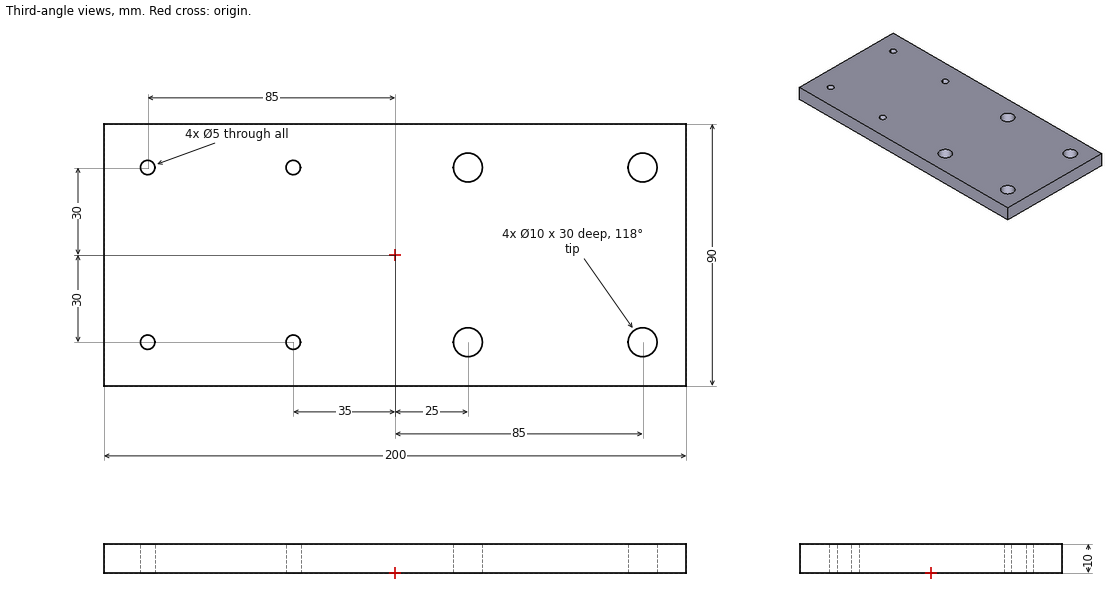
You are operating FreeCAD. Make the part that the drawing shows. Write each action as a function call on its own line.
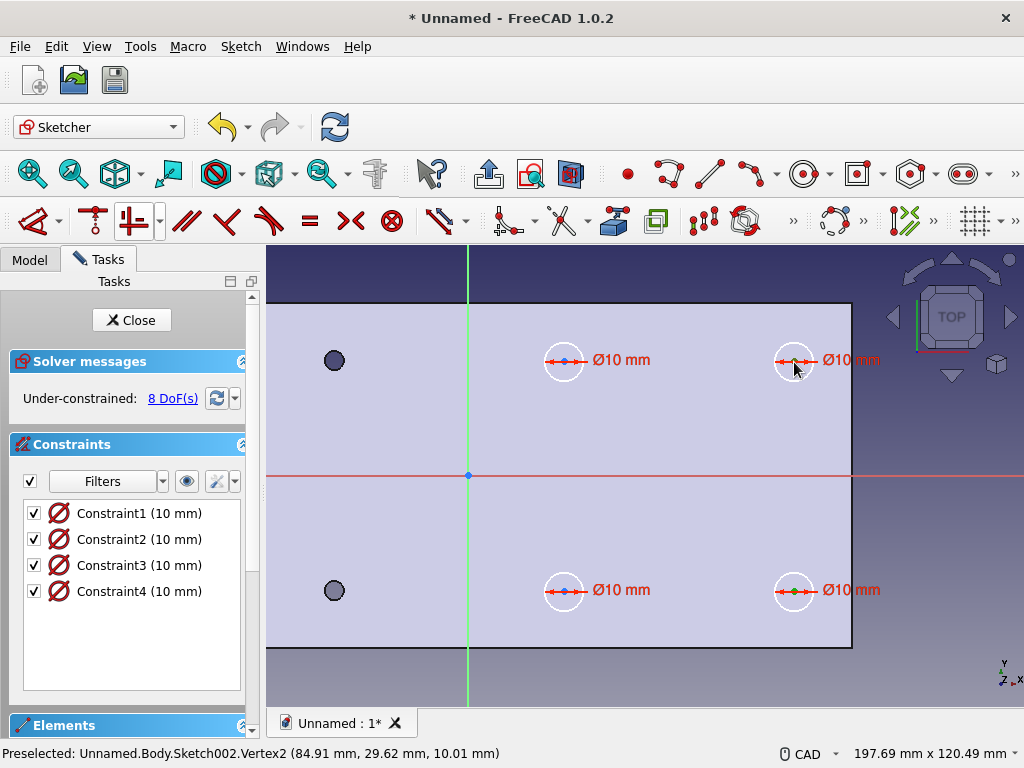
key(v)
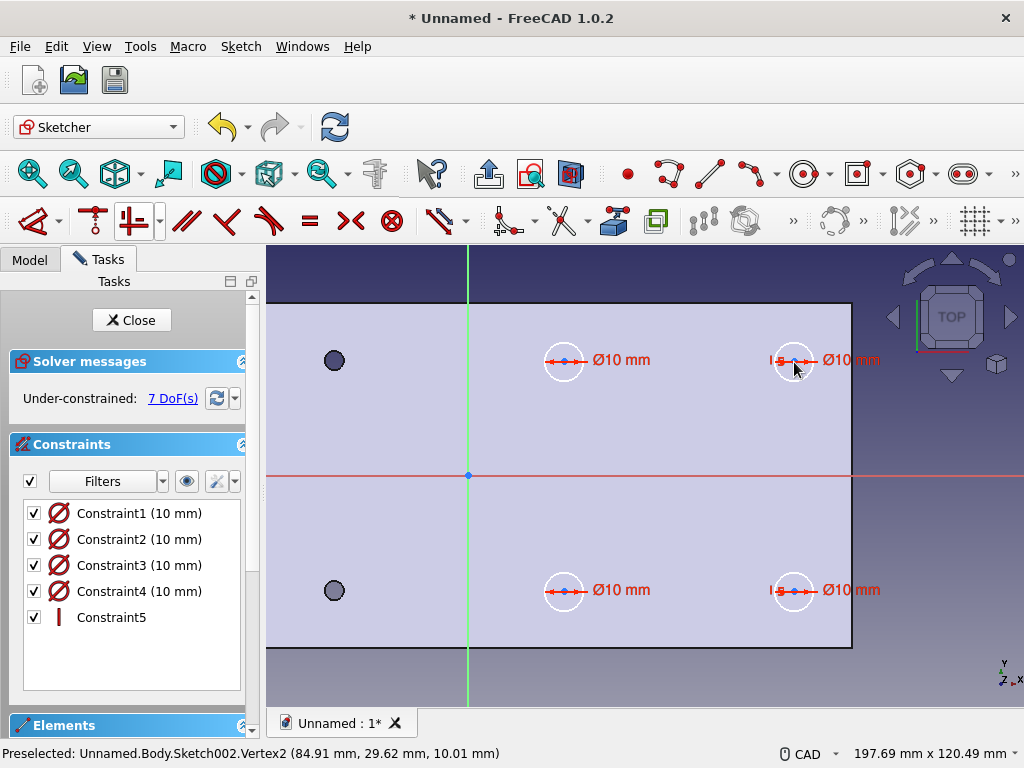
click(794, 592)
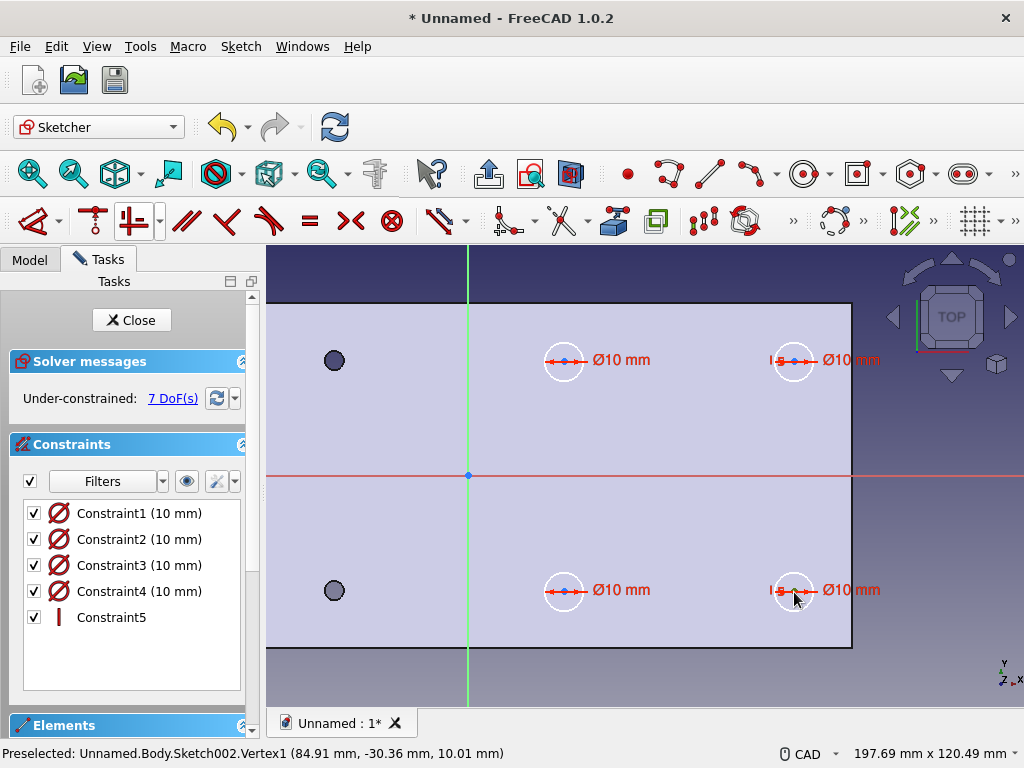
click(564, 592)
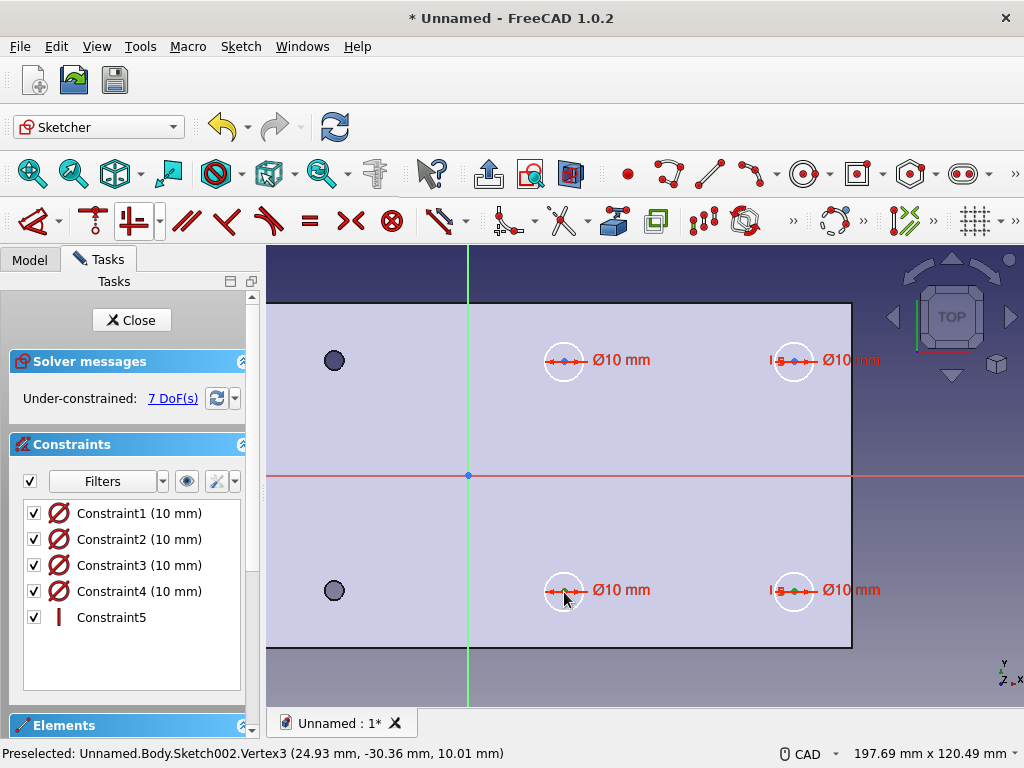
key(h)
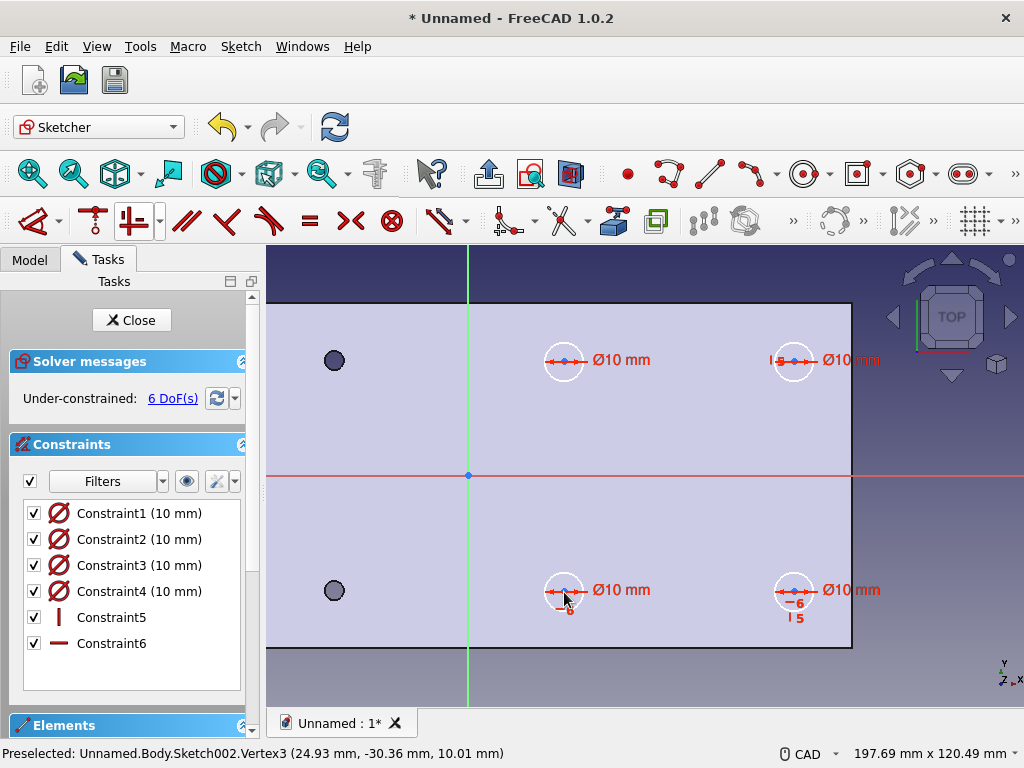
click(564, 592)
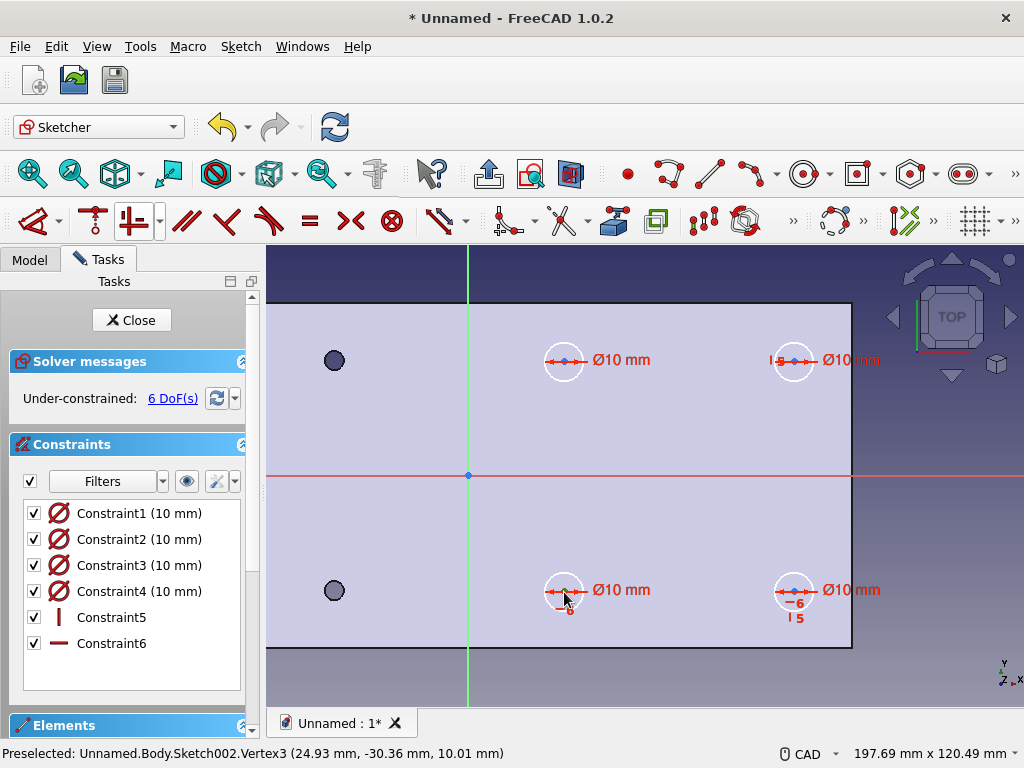
click(564, 362)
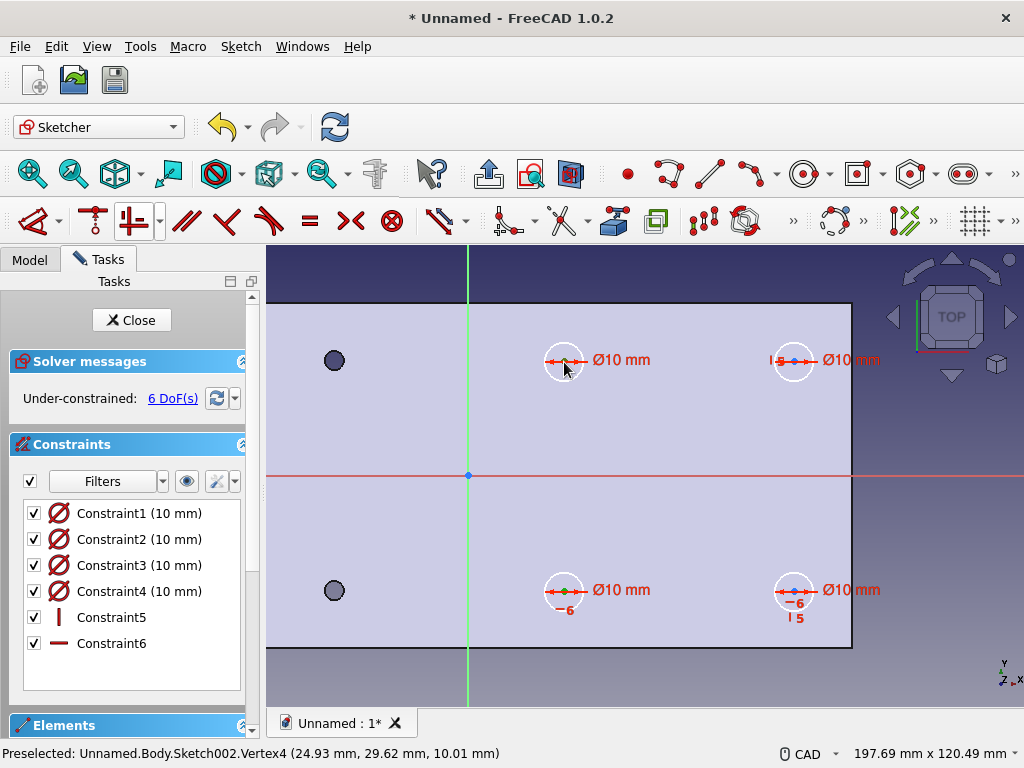
key(v)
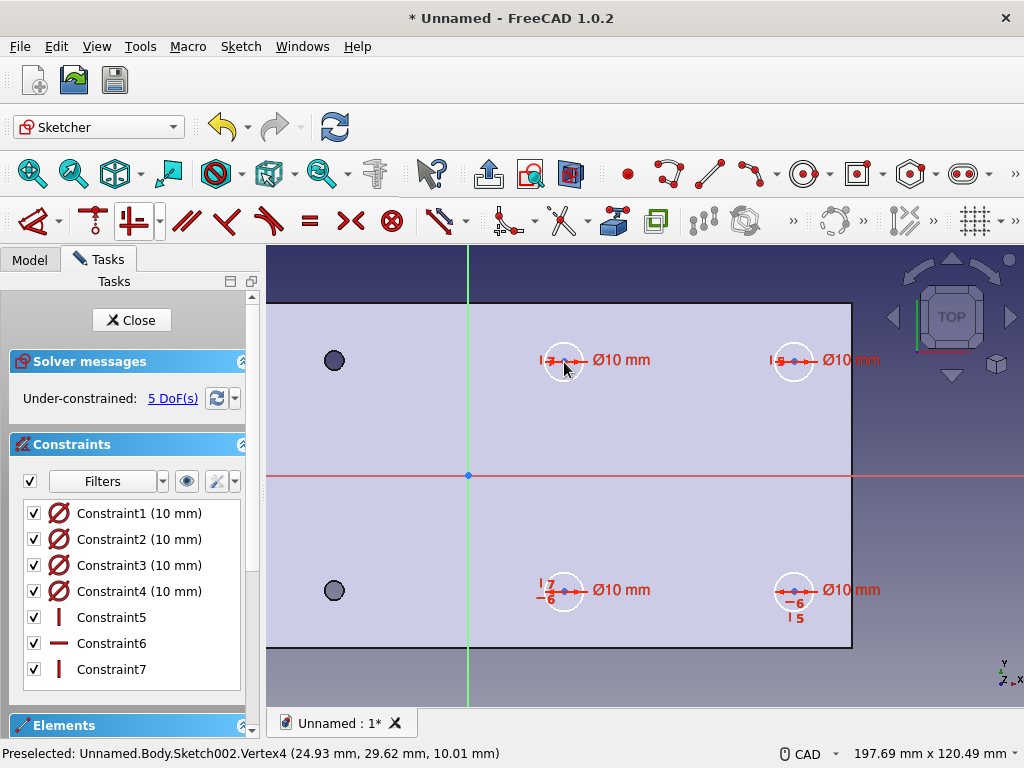
click(794, 362)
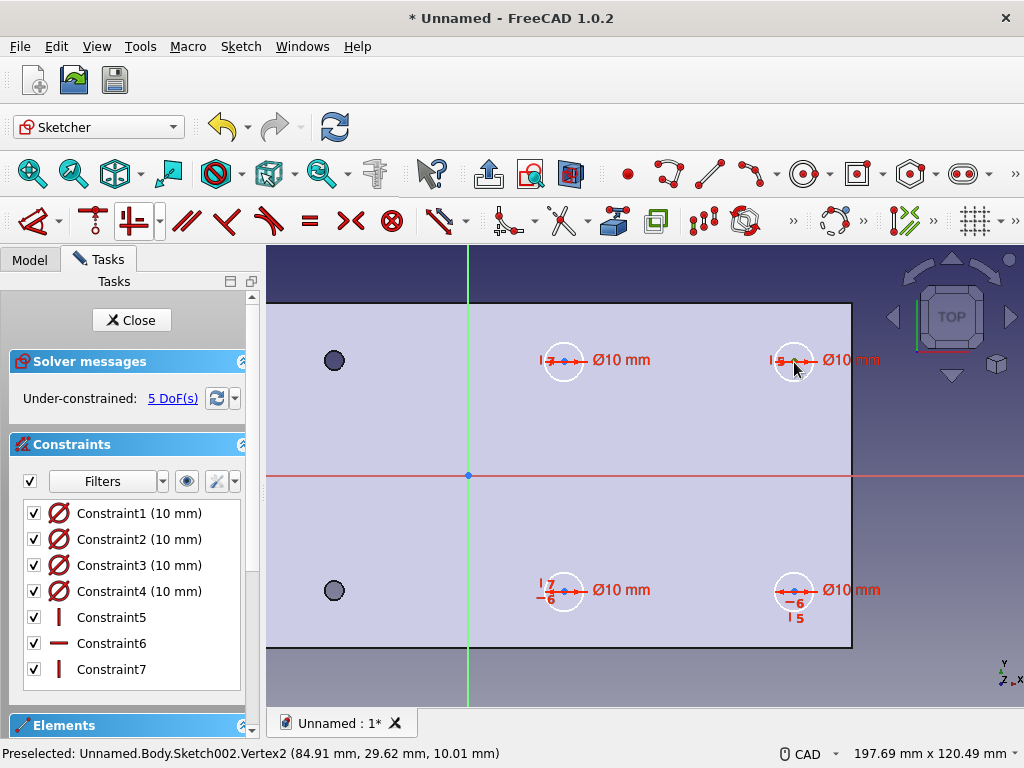
click(564, 362)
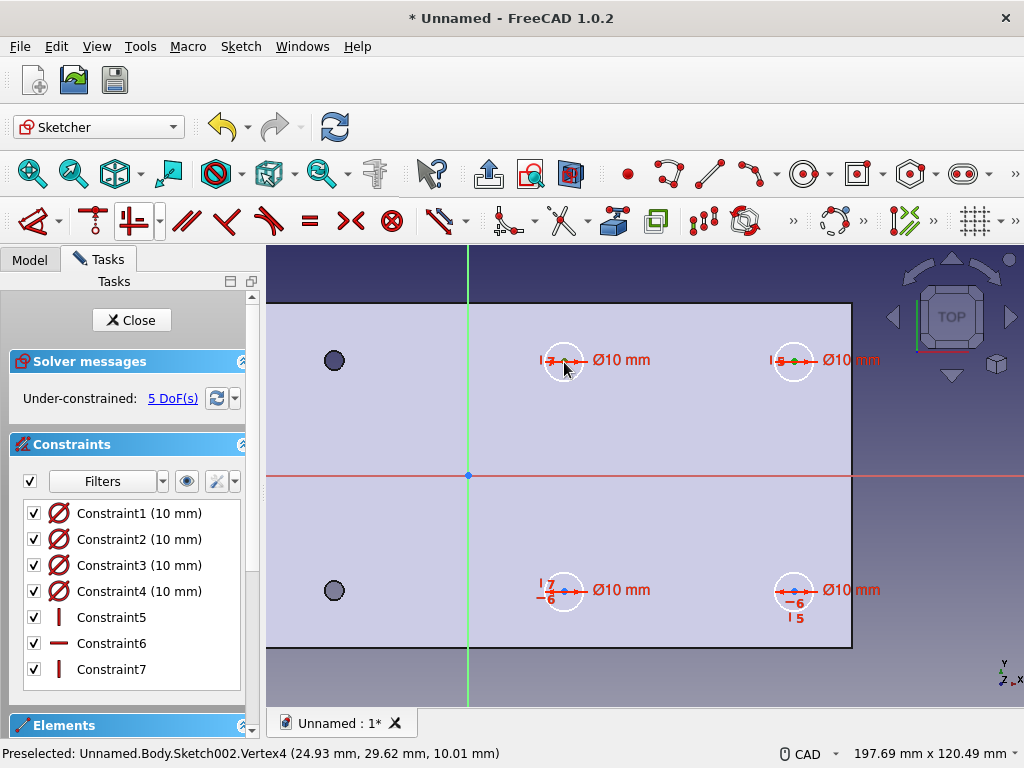
click(160, 222)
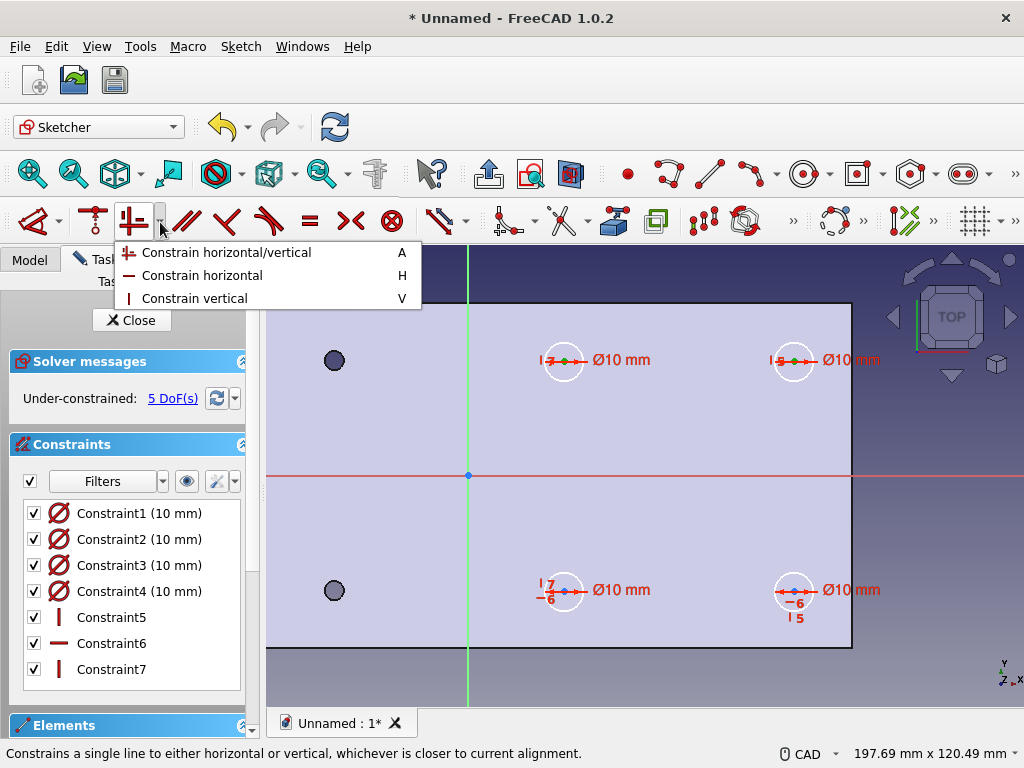
click(268, 276)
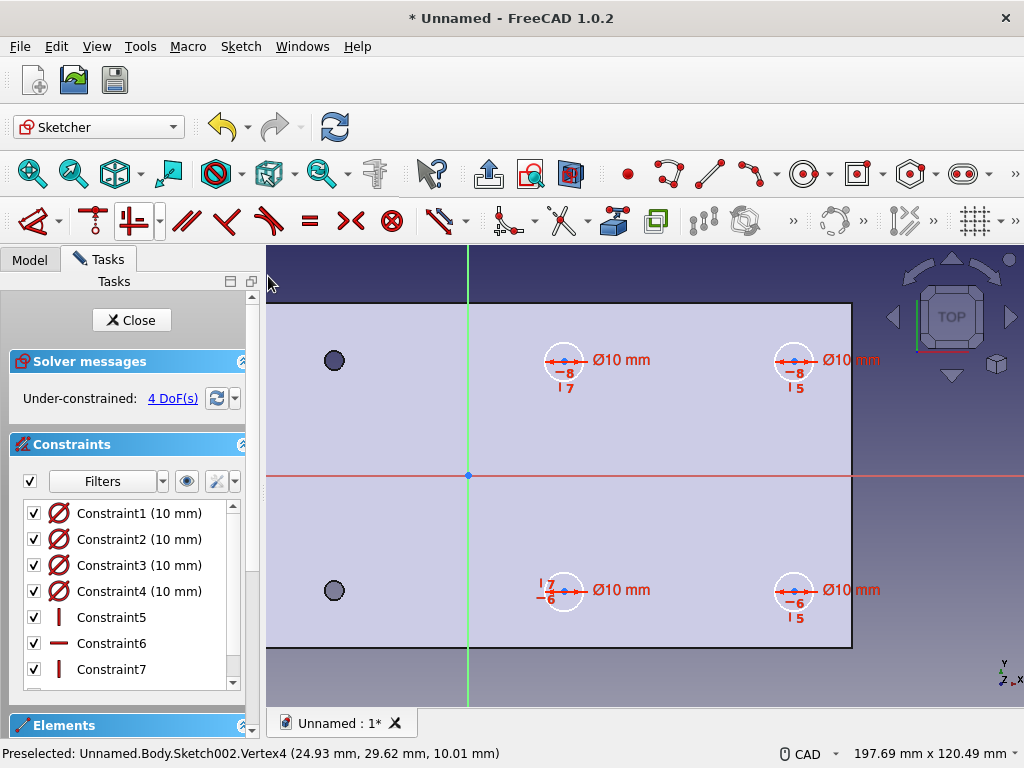
click(32, 222)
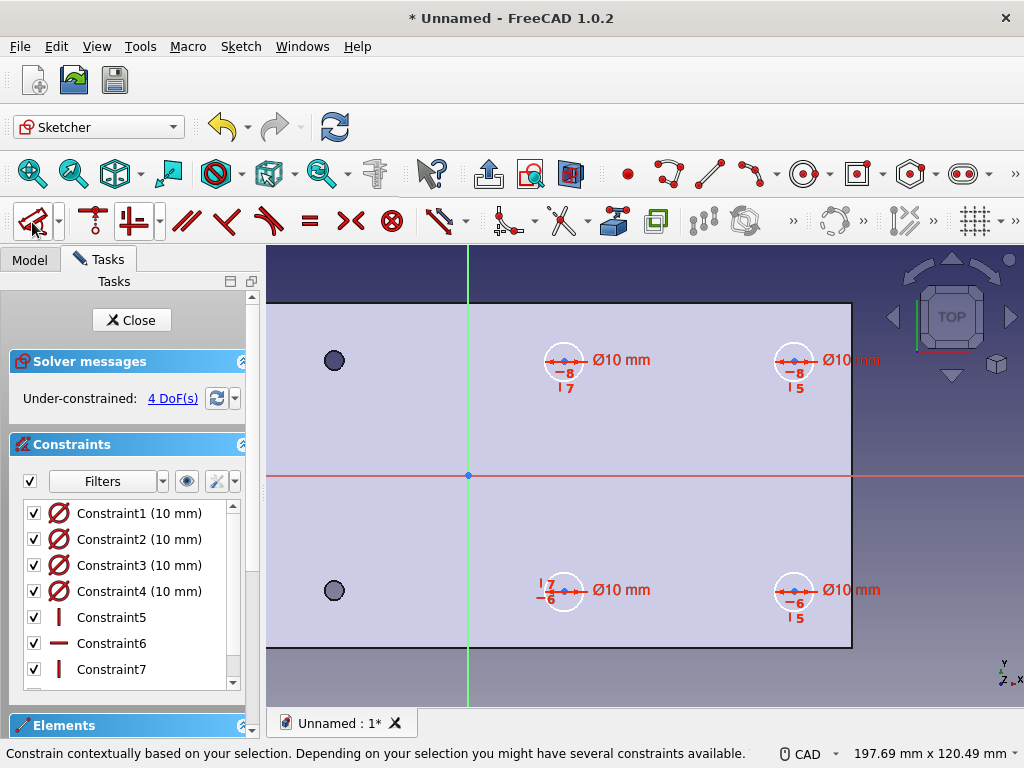
click(794, 592)
click(631, 626)